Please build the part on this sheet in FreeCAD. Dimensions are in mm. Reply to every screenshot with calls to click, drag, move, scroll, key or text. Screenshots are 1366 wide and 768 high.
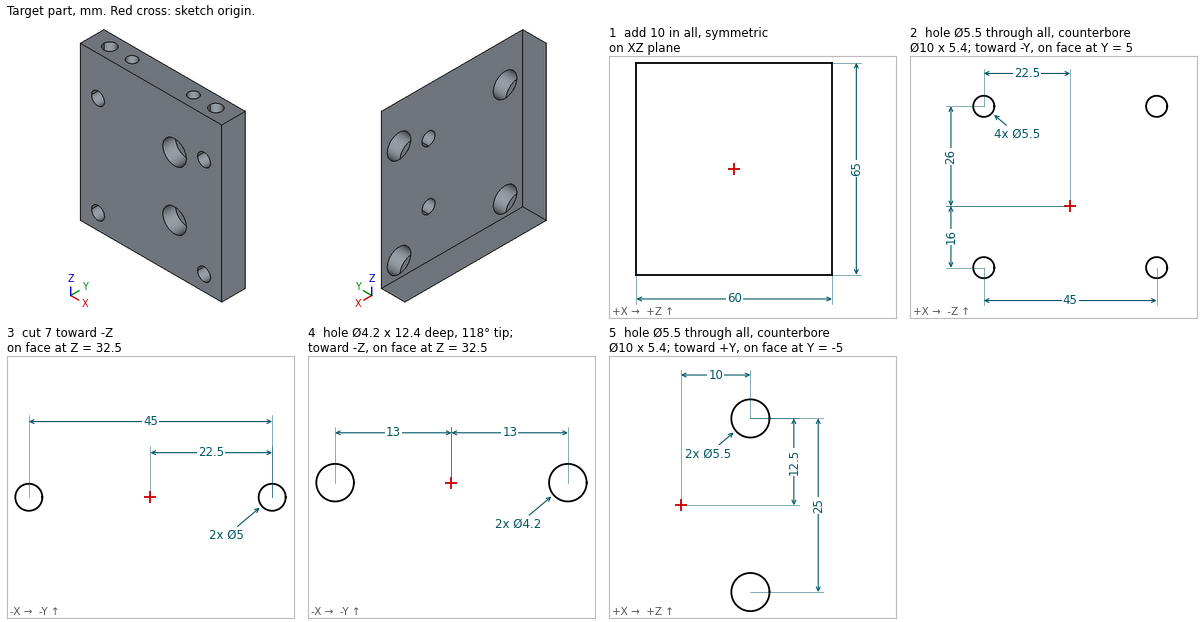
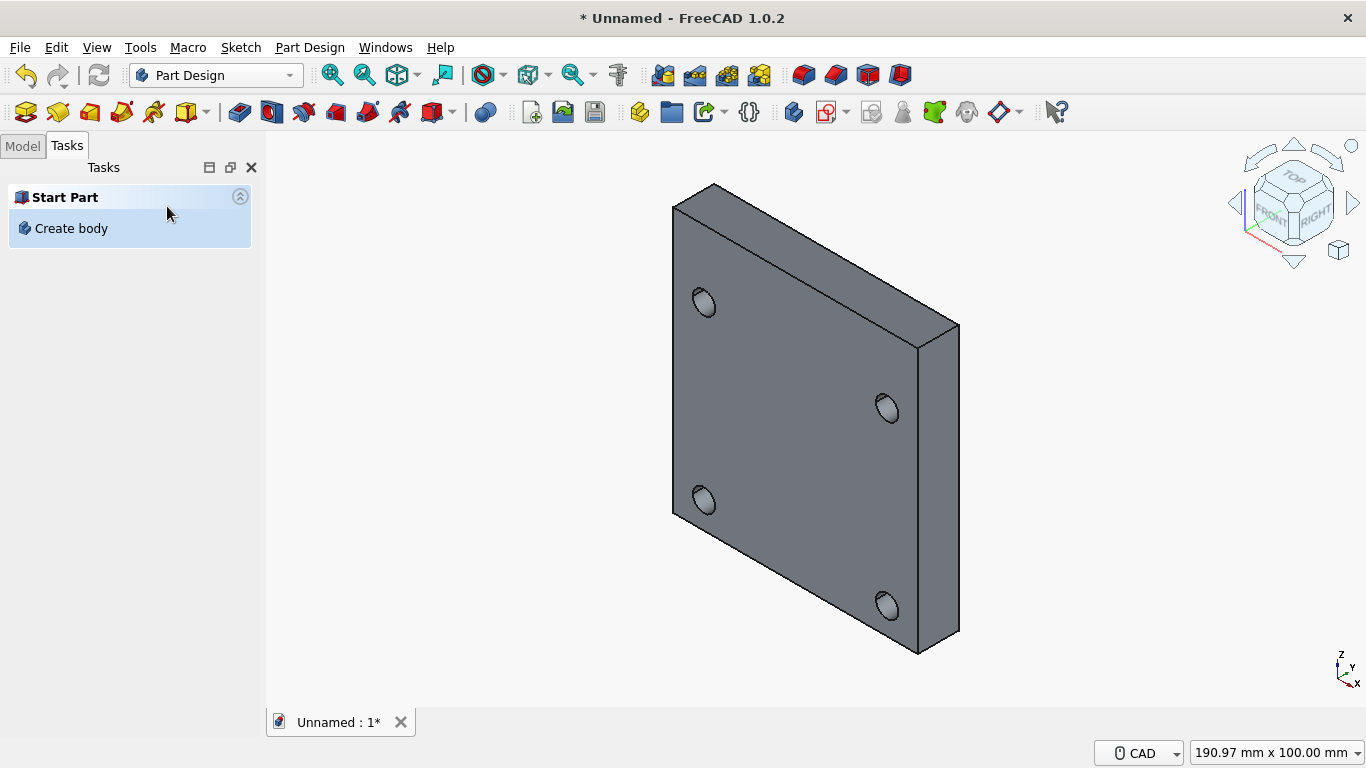
click(886, 305)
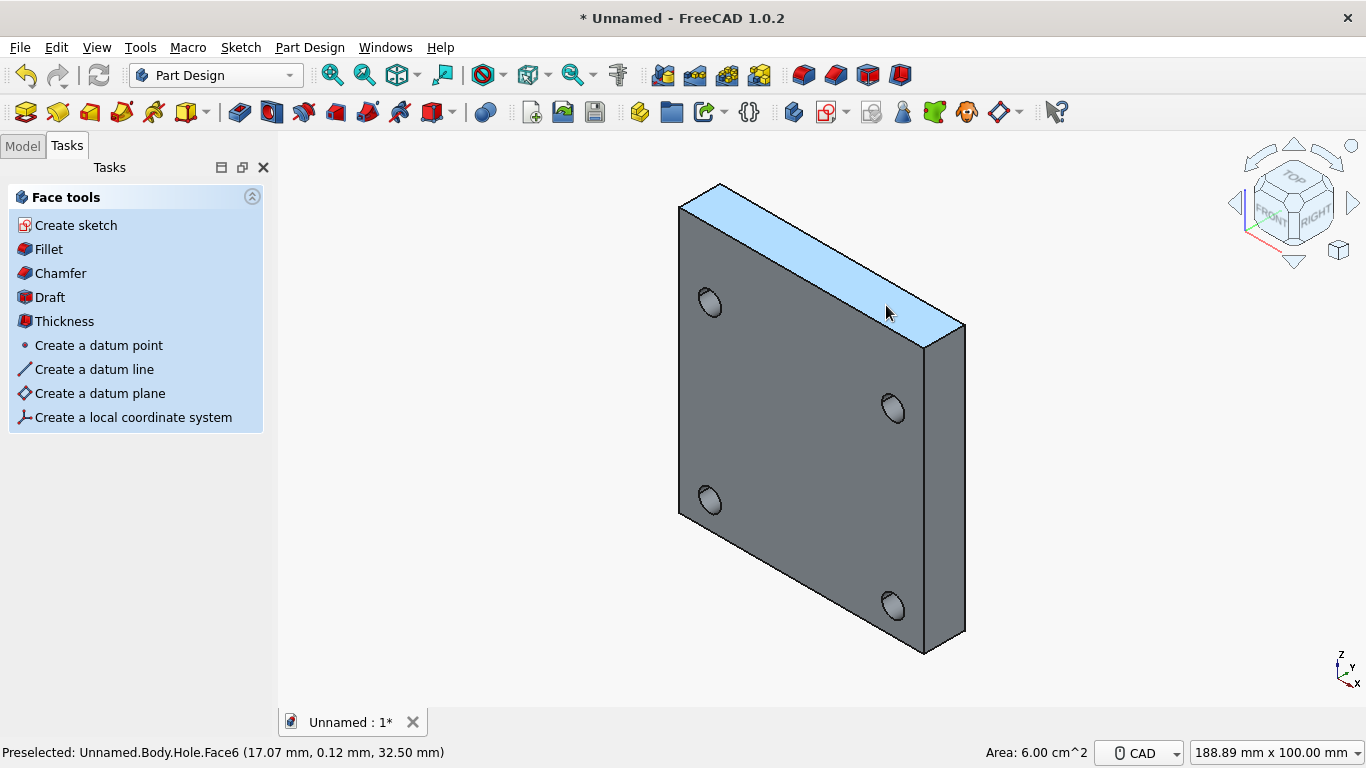
click(826, 112)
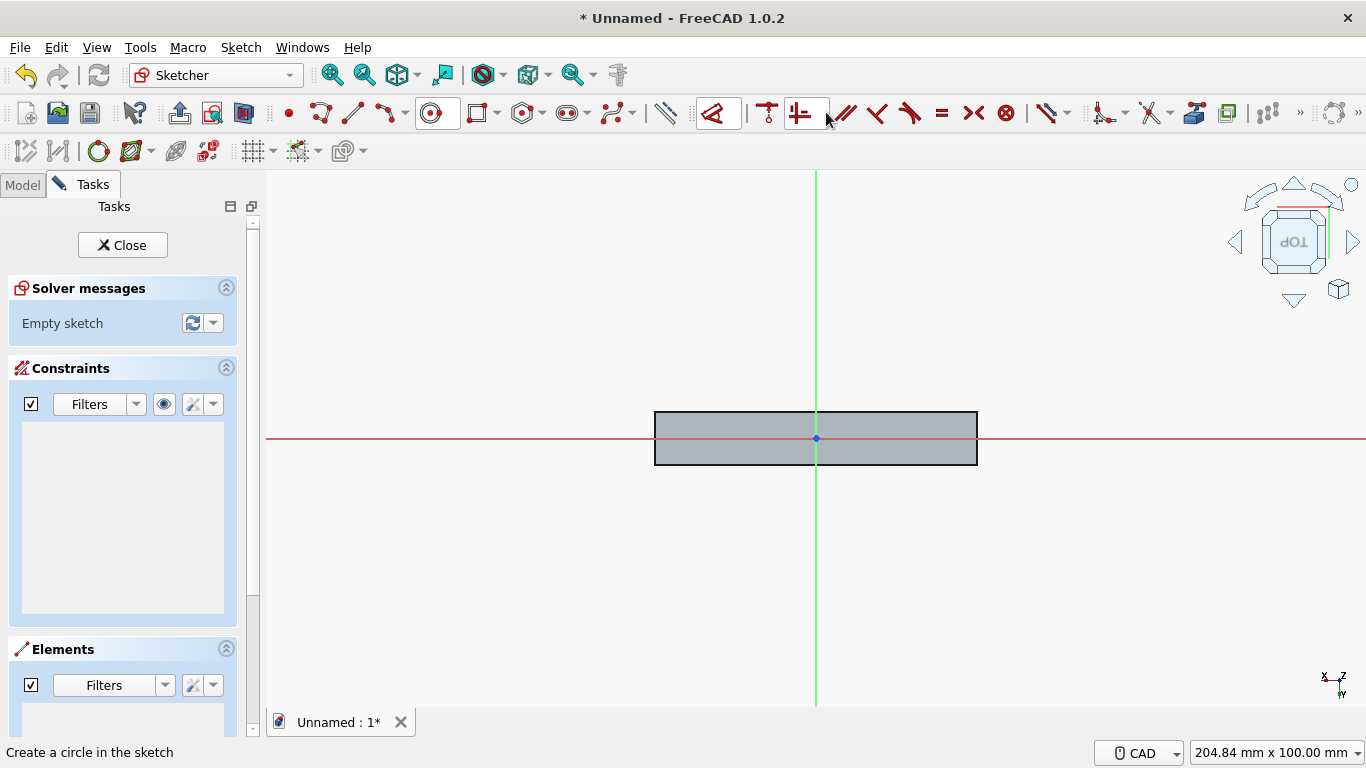
scroll(872, 439, up, 4)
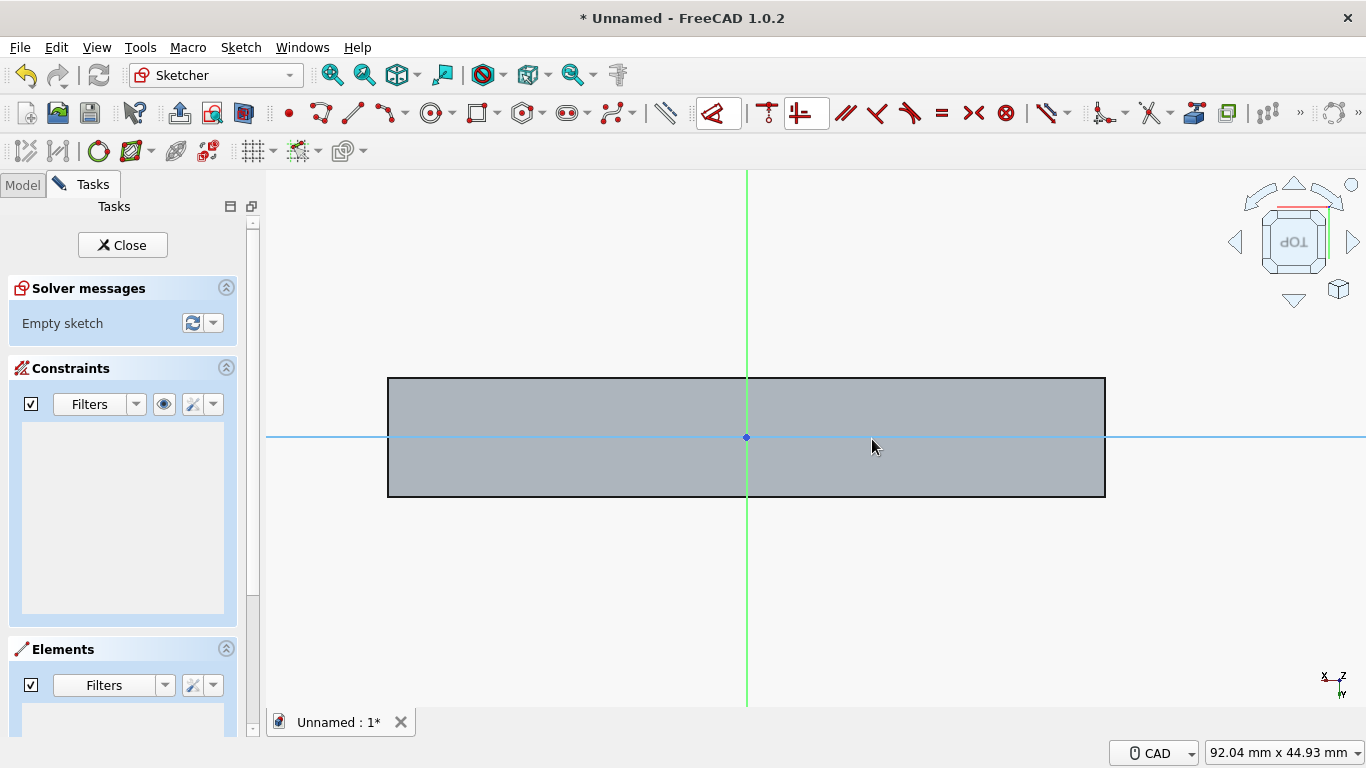
click(432, 114)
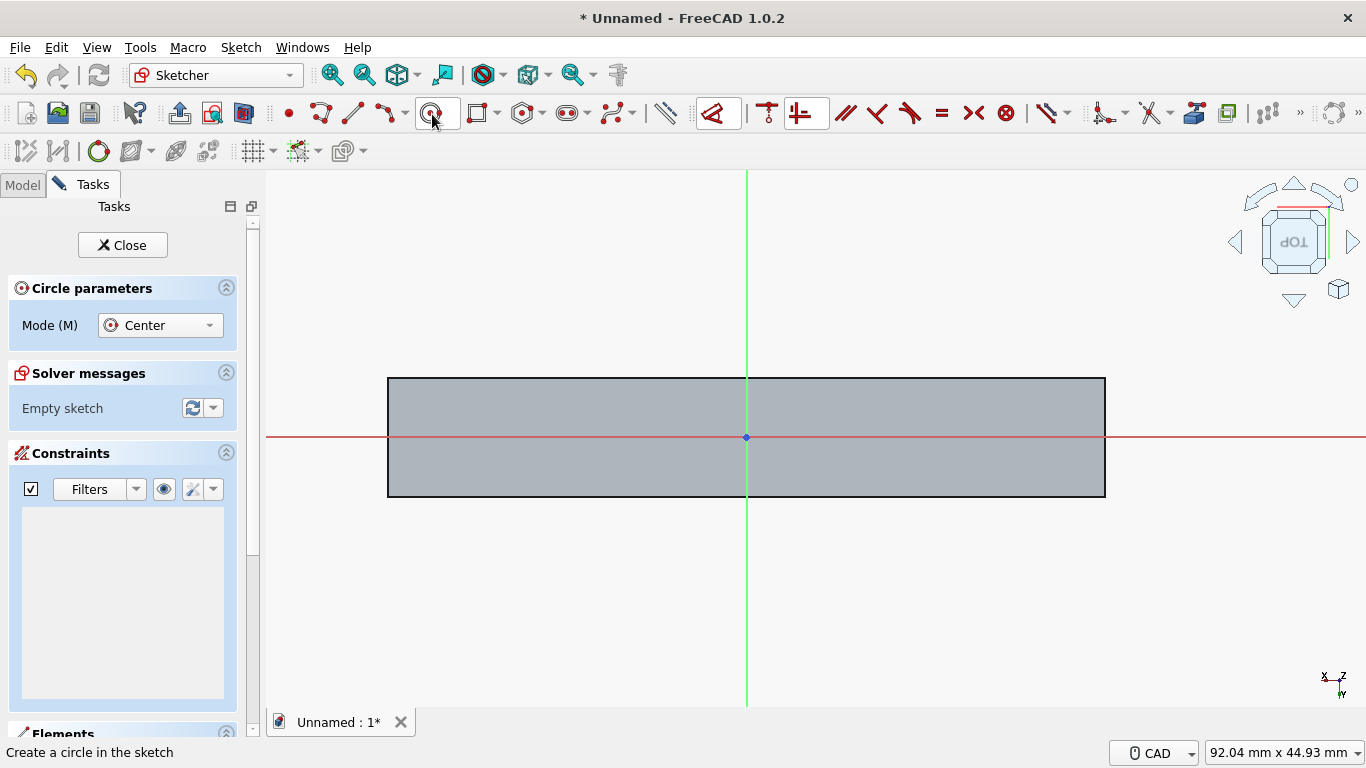
click(1016, 437)
click(1037, 416)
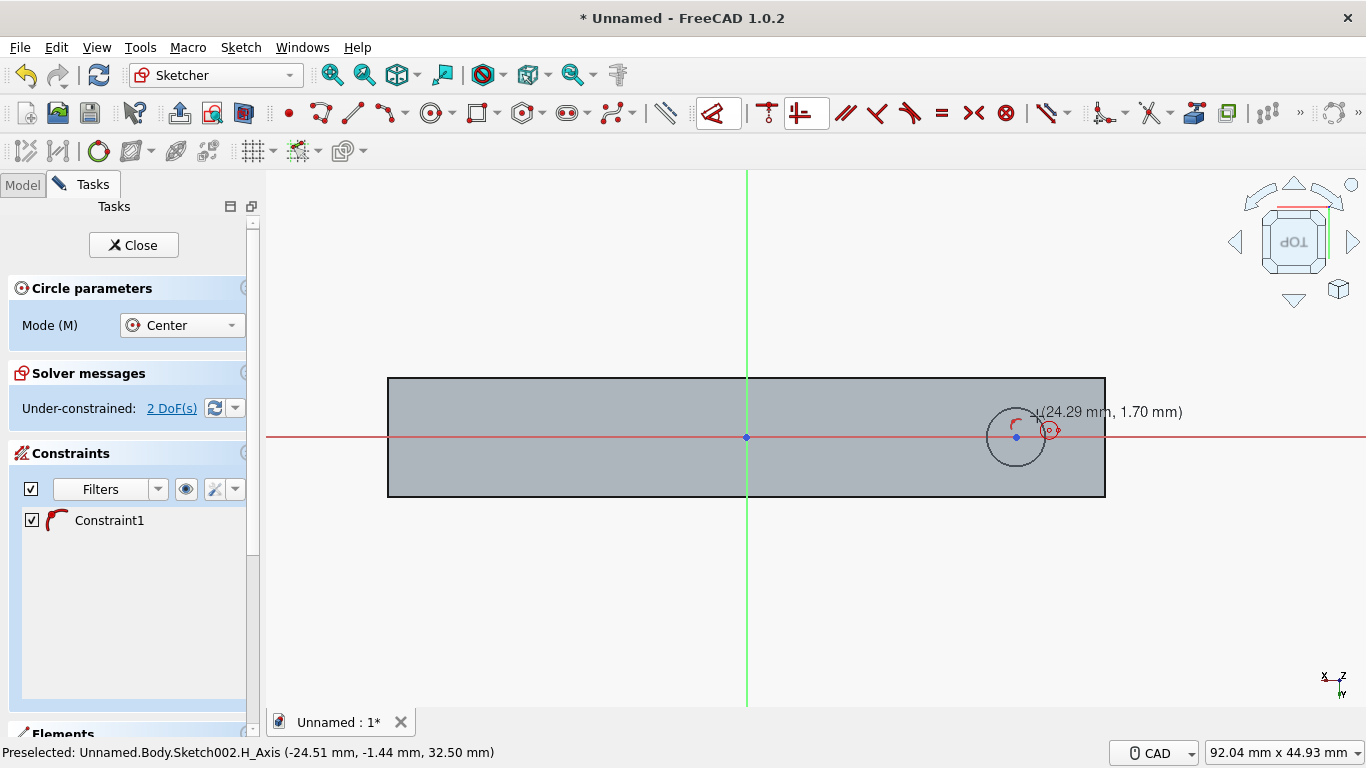
click(478, 437)
click(499, 416)
key(Escape)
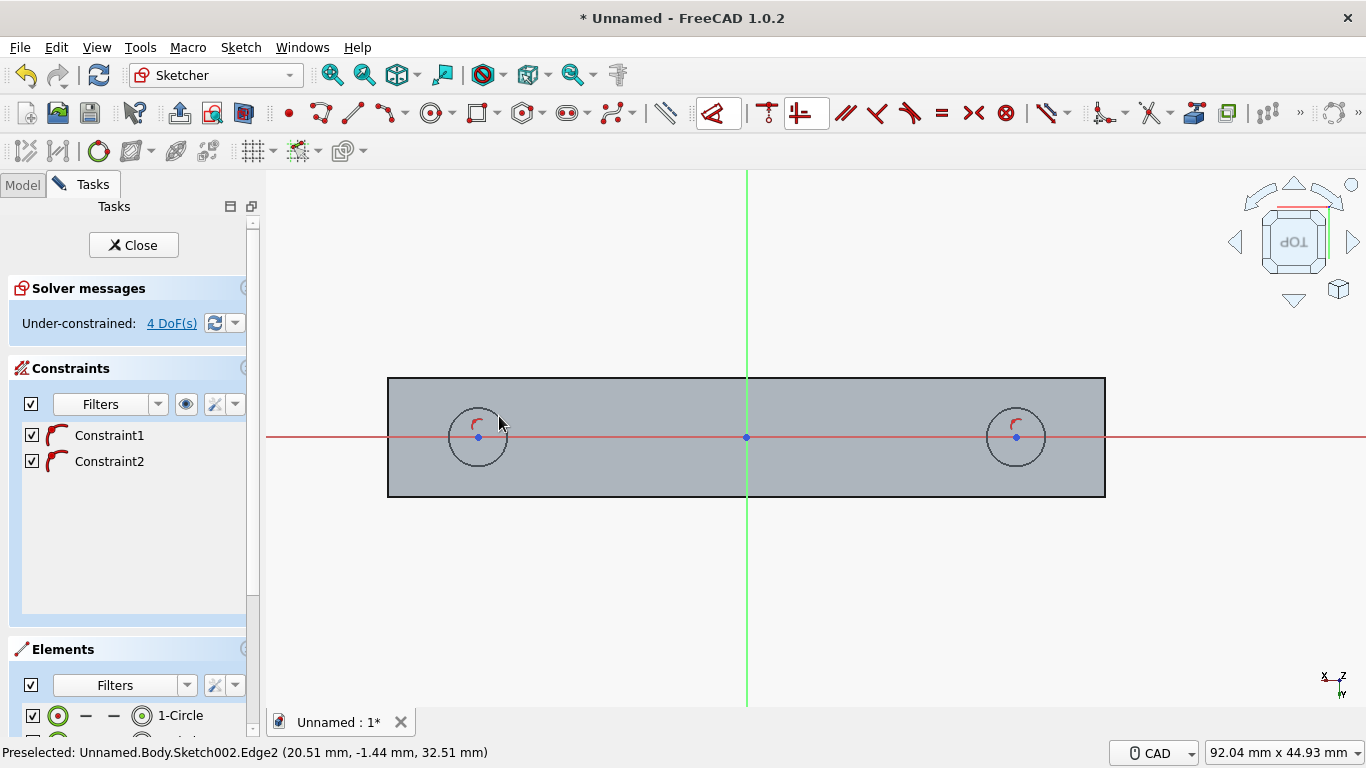
click(1037, 417)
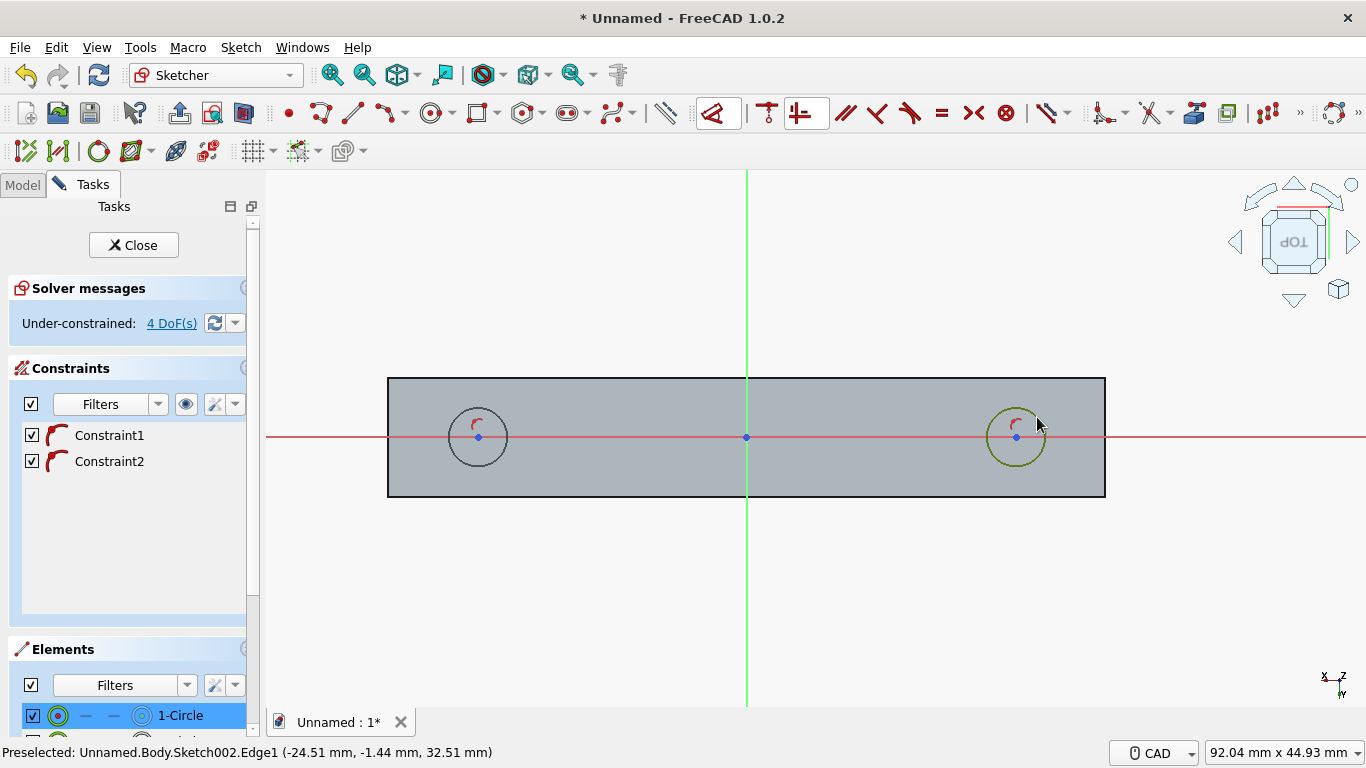
click(499, 417)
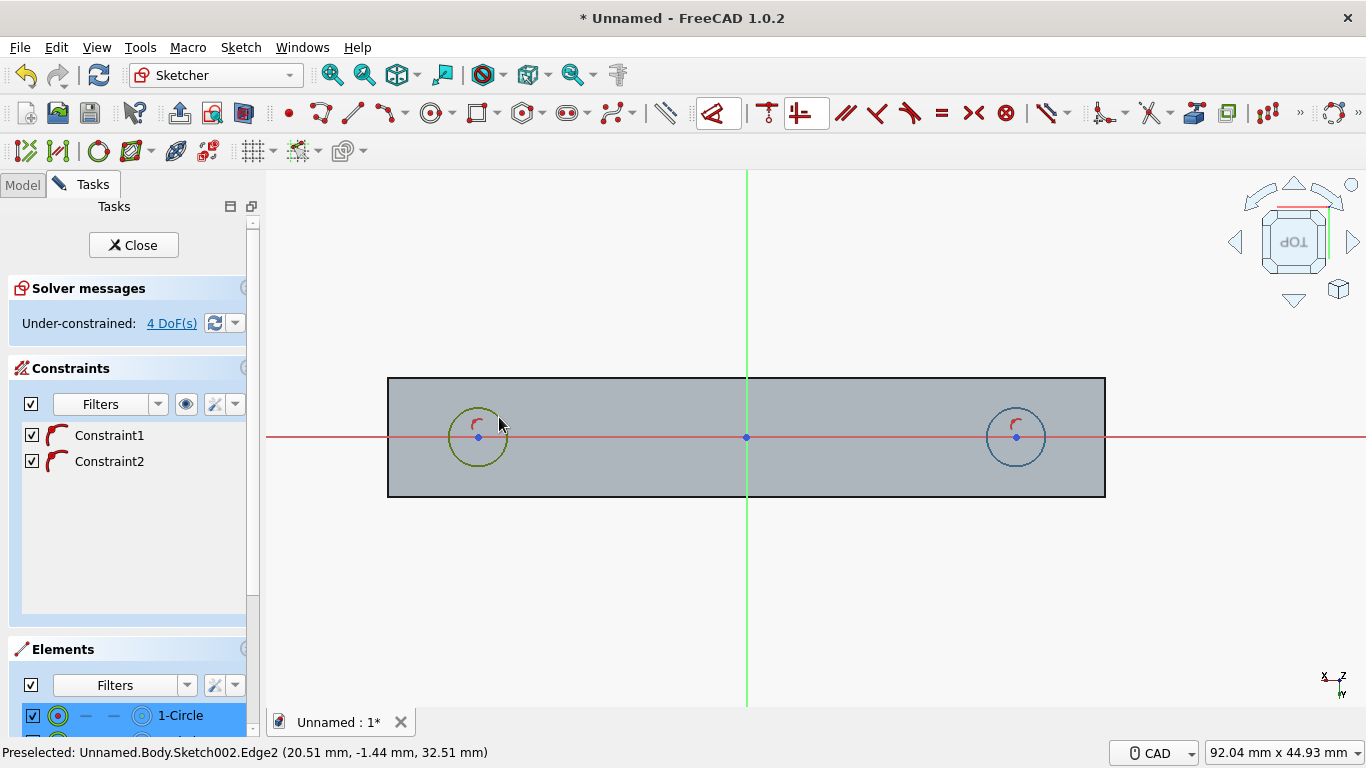
click(942, 114)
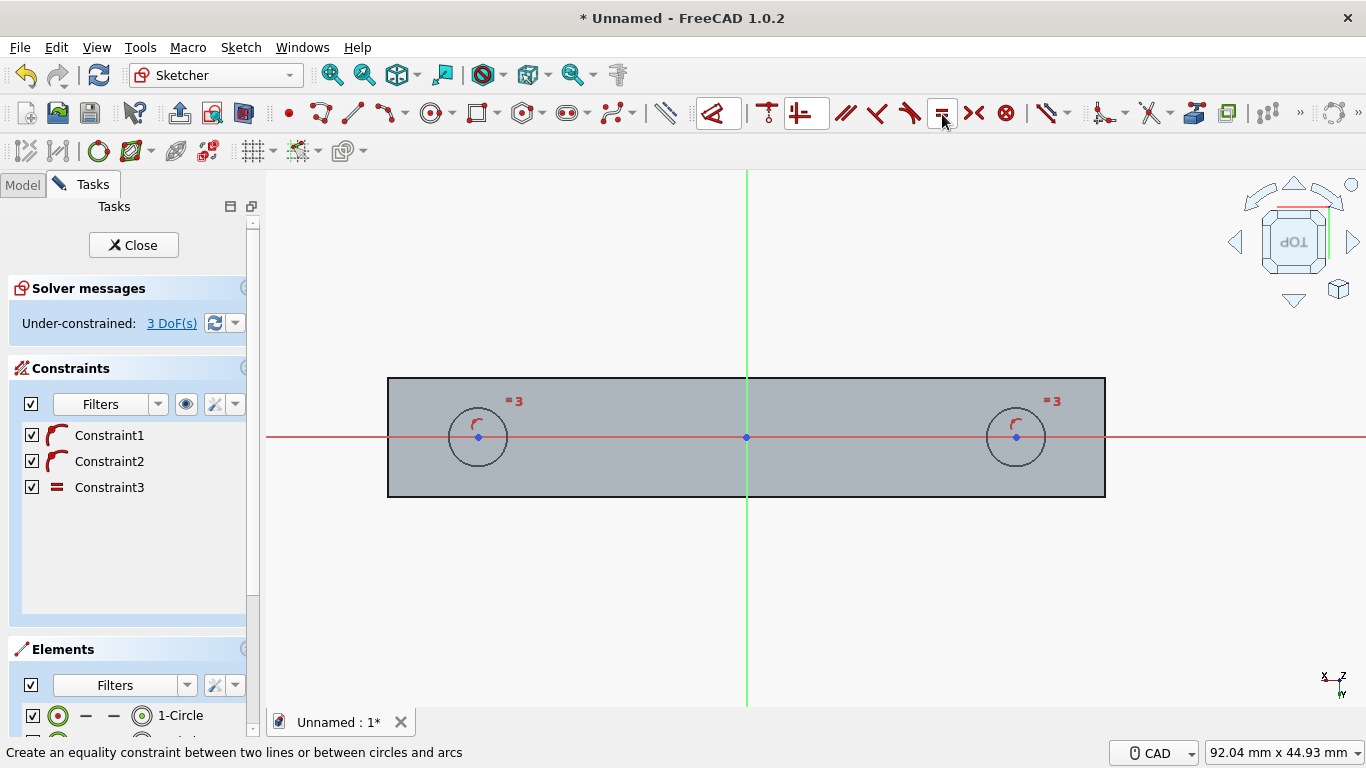
click(1037, 417)